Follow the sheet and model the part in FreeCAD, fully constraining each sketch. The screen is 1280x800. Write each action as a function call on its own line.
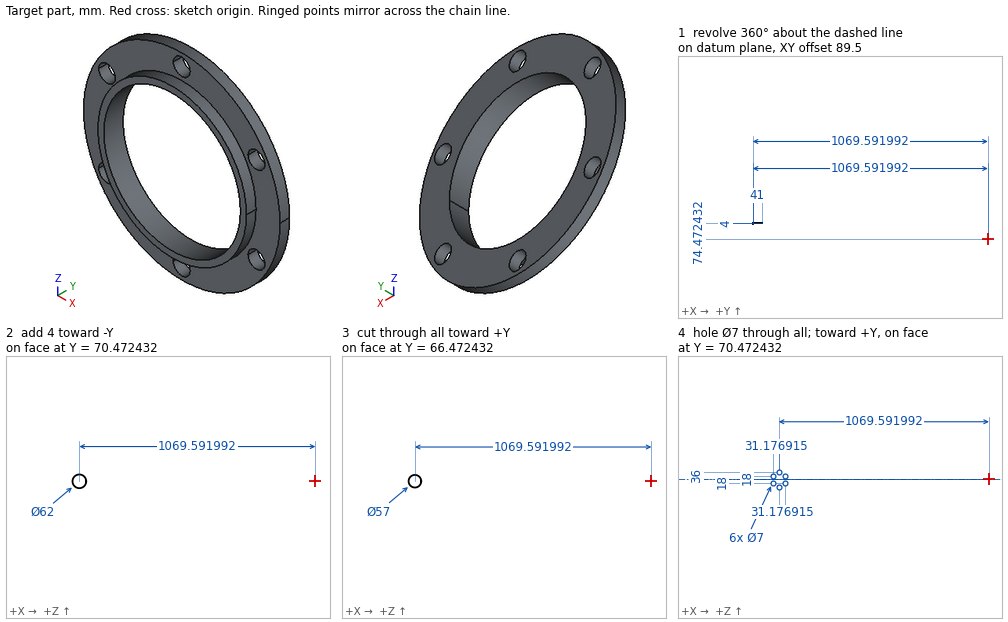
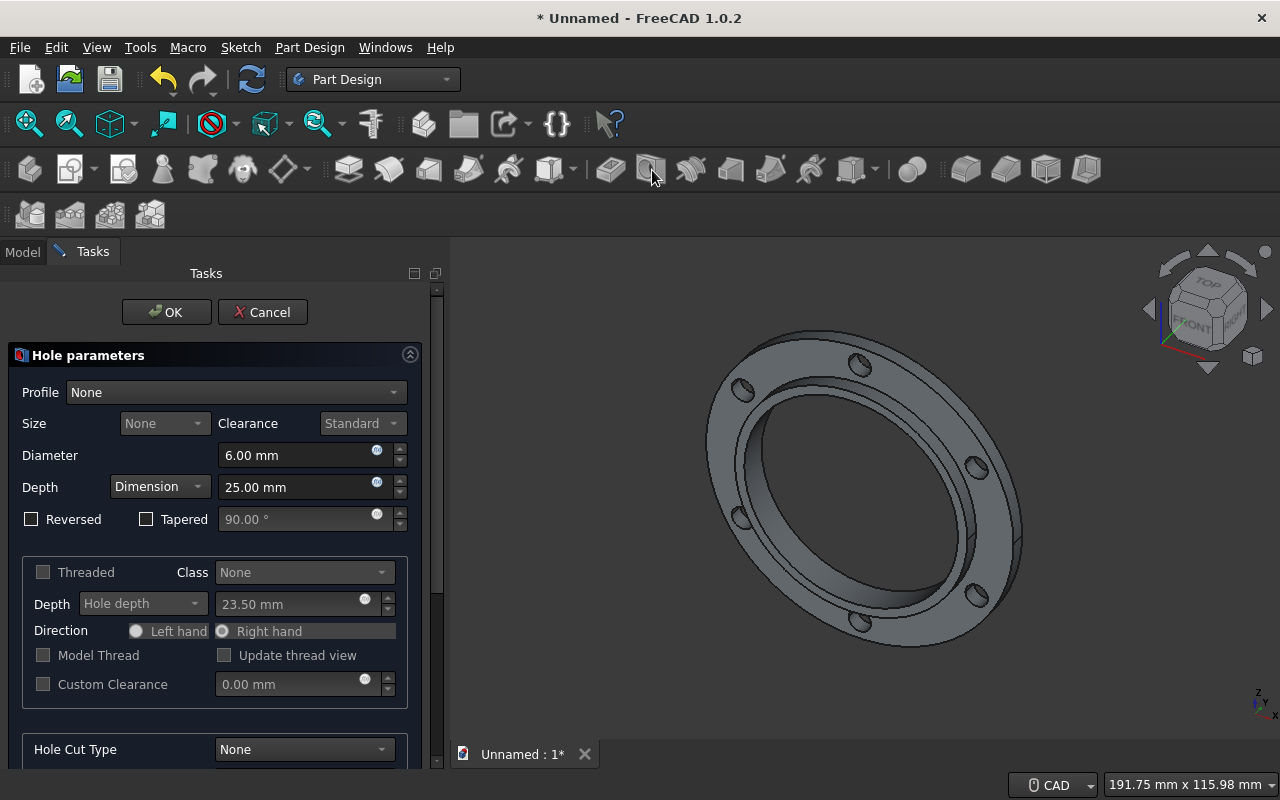
triple_click(305, 455)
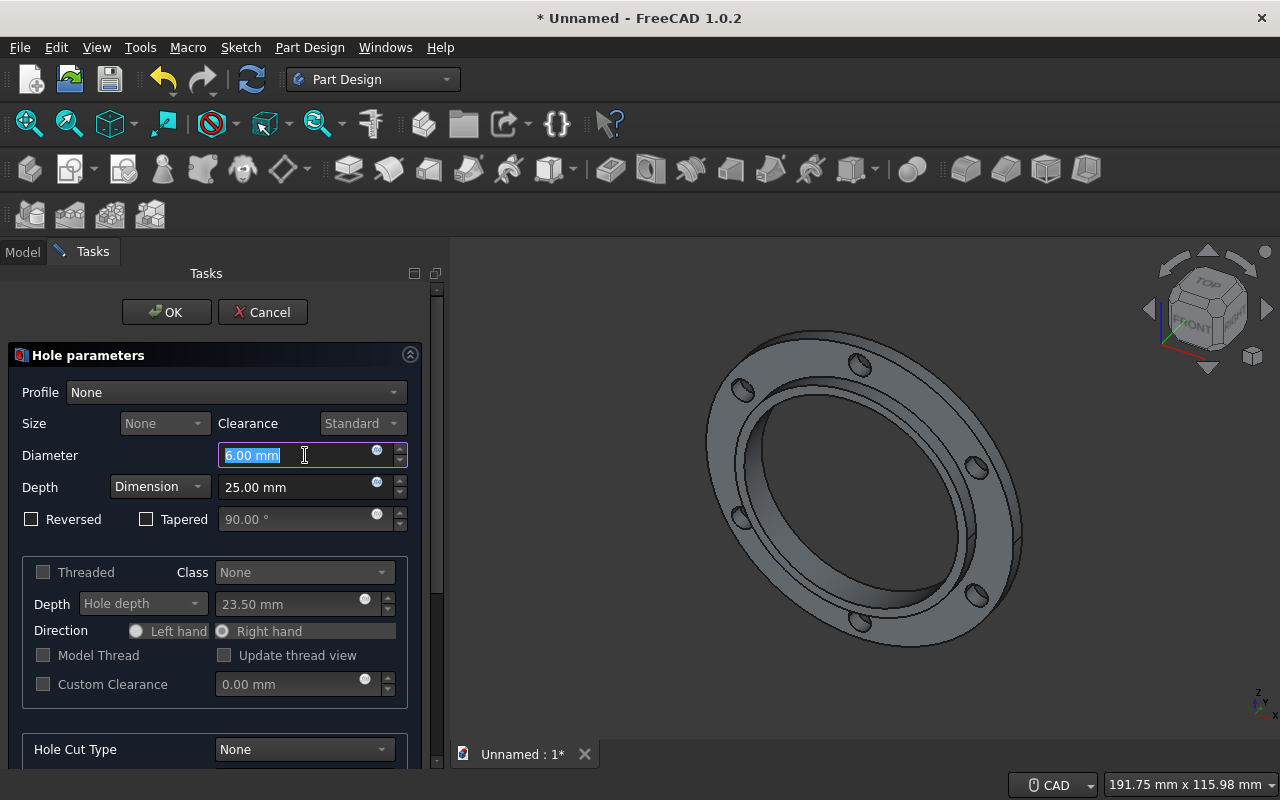
text(7)
key(Tab)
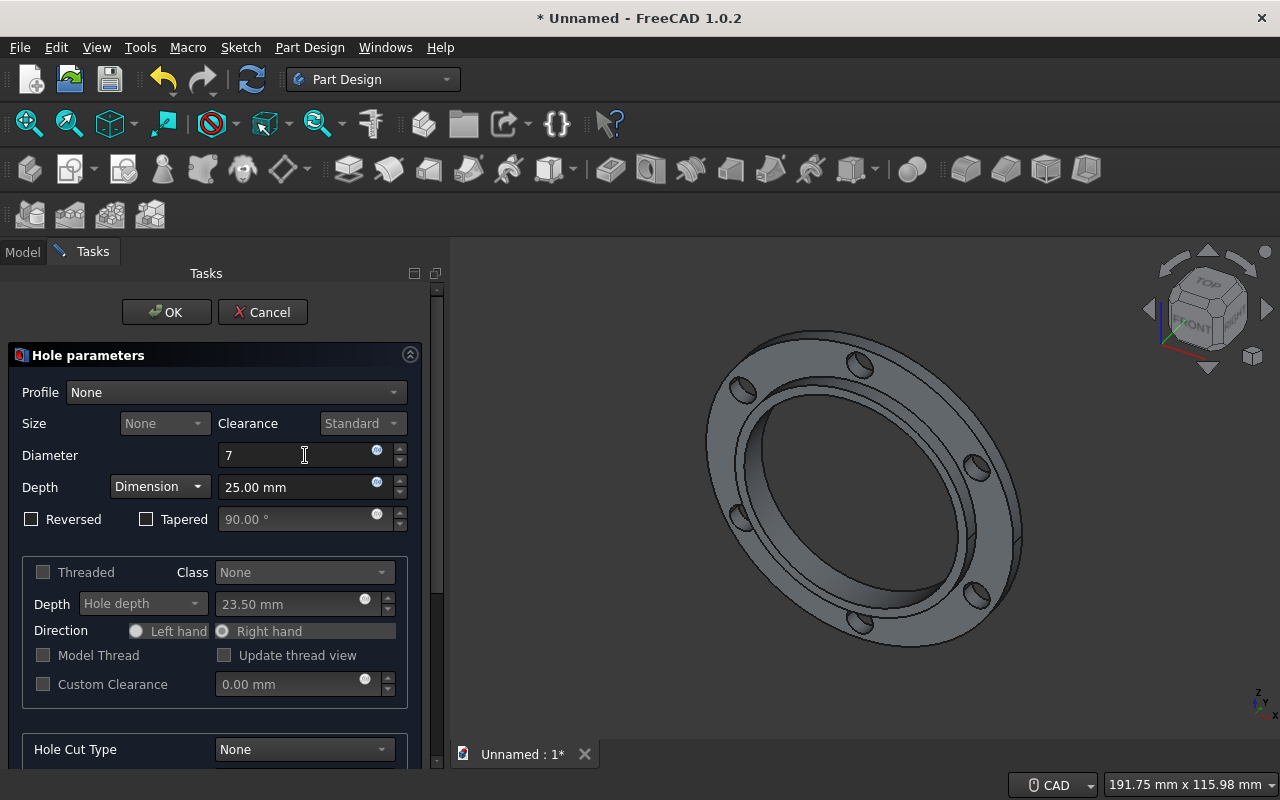
click(161, 486)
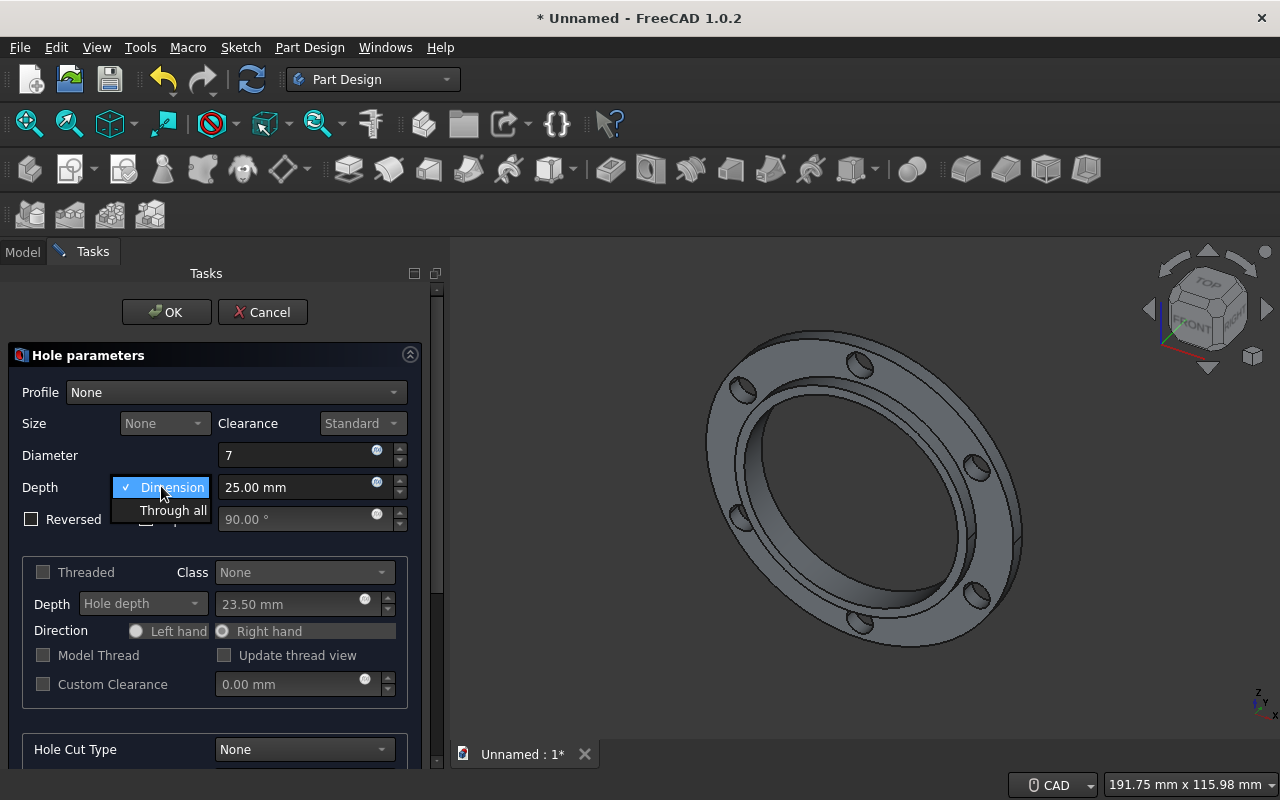
click(160, 510)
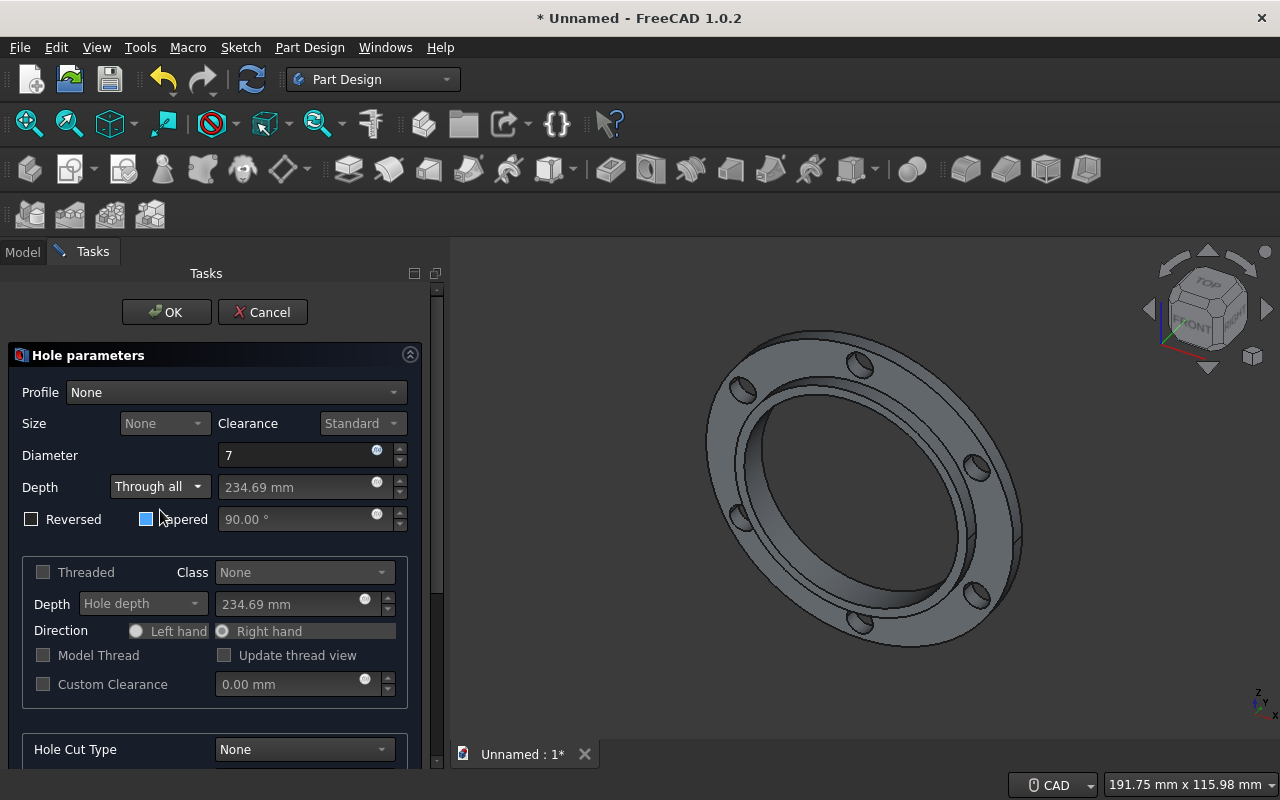
click(167, 312)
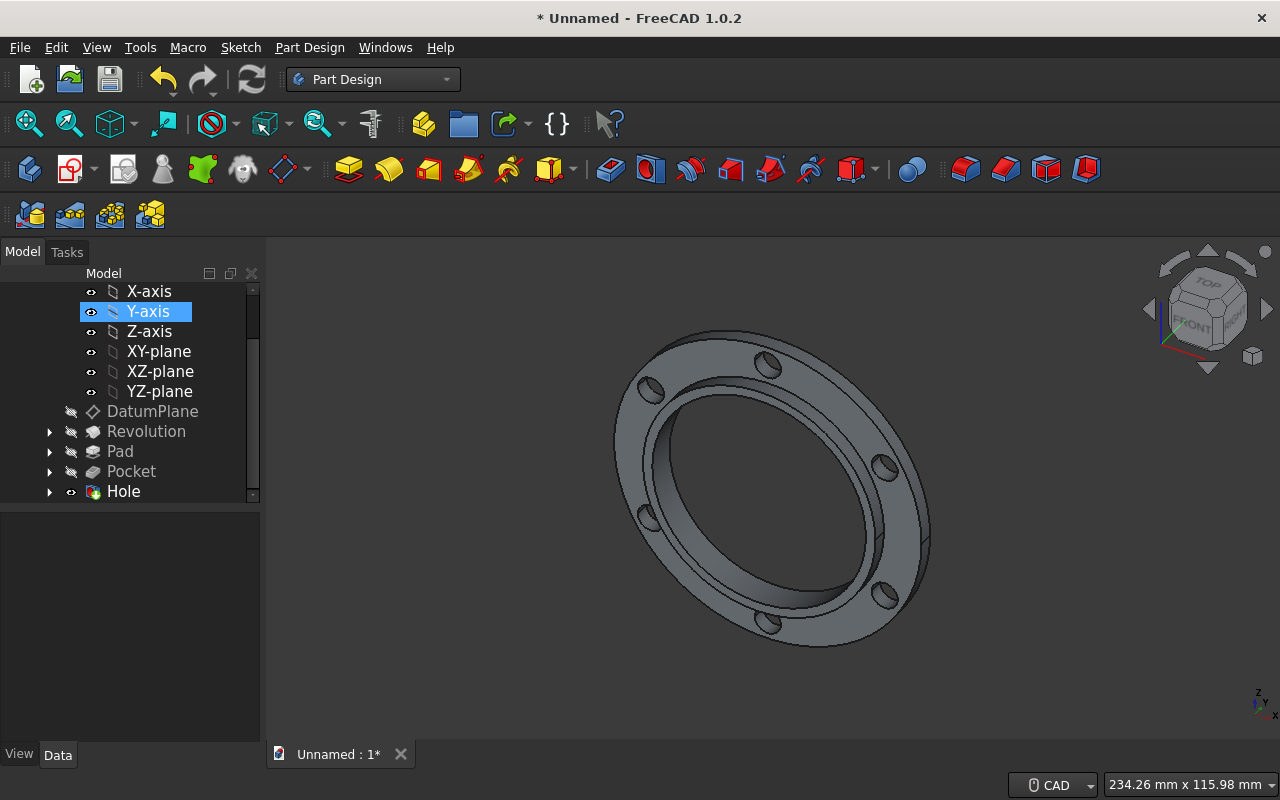
key(0)